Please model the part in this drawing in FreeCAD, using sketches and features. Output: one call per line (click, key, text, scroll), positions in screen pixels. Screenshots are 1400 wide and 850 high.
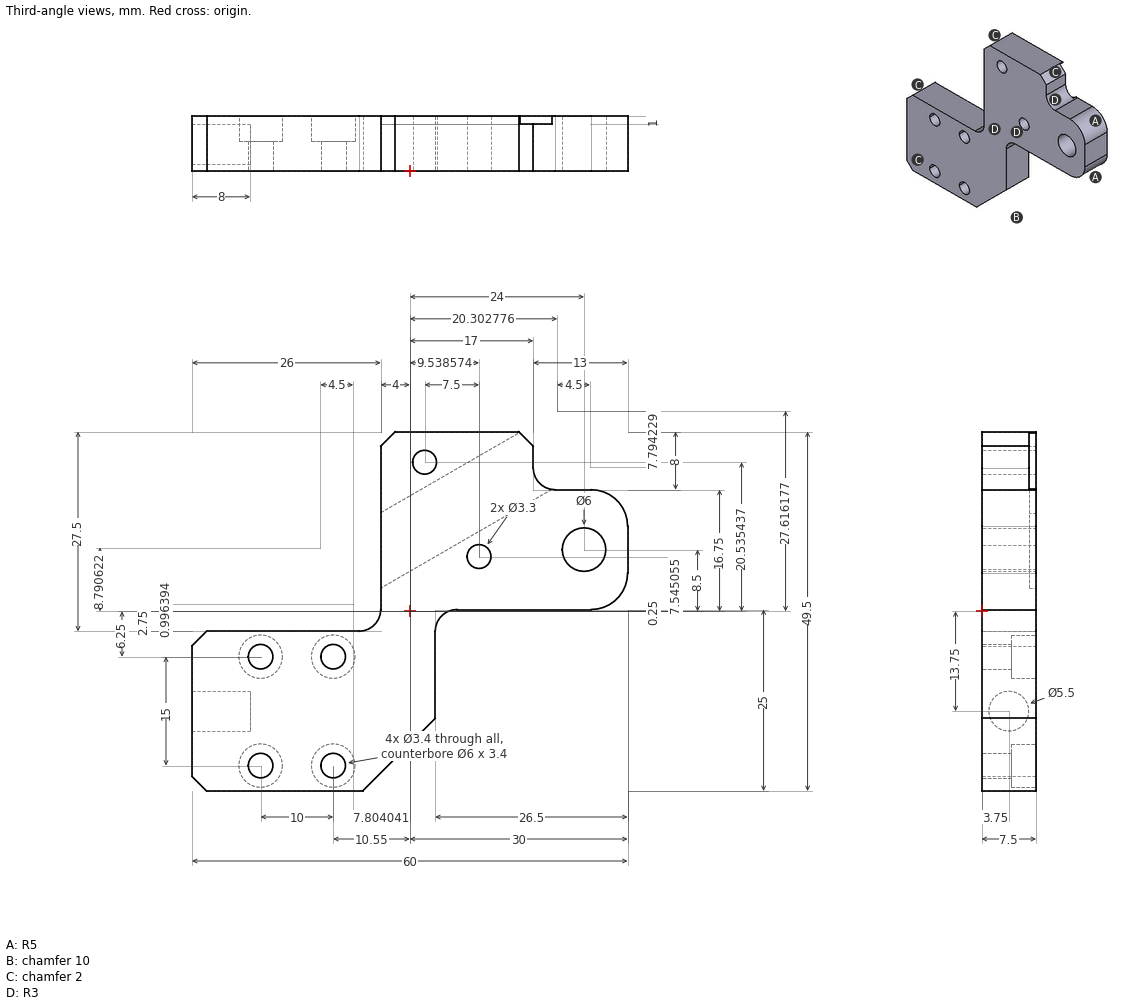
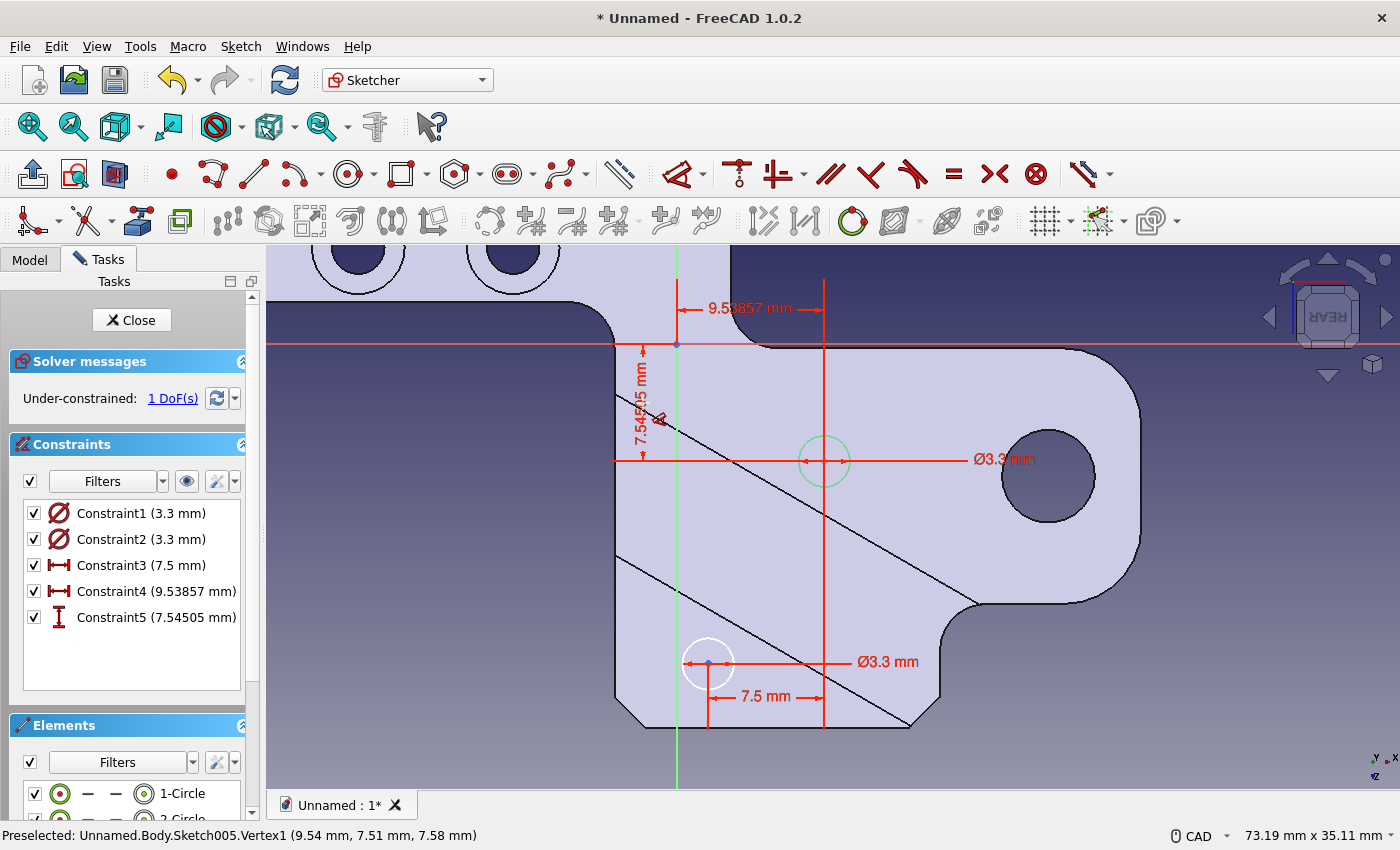
click(708, 664)
click(643, 504)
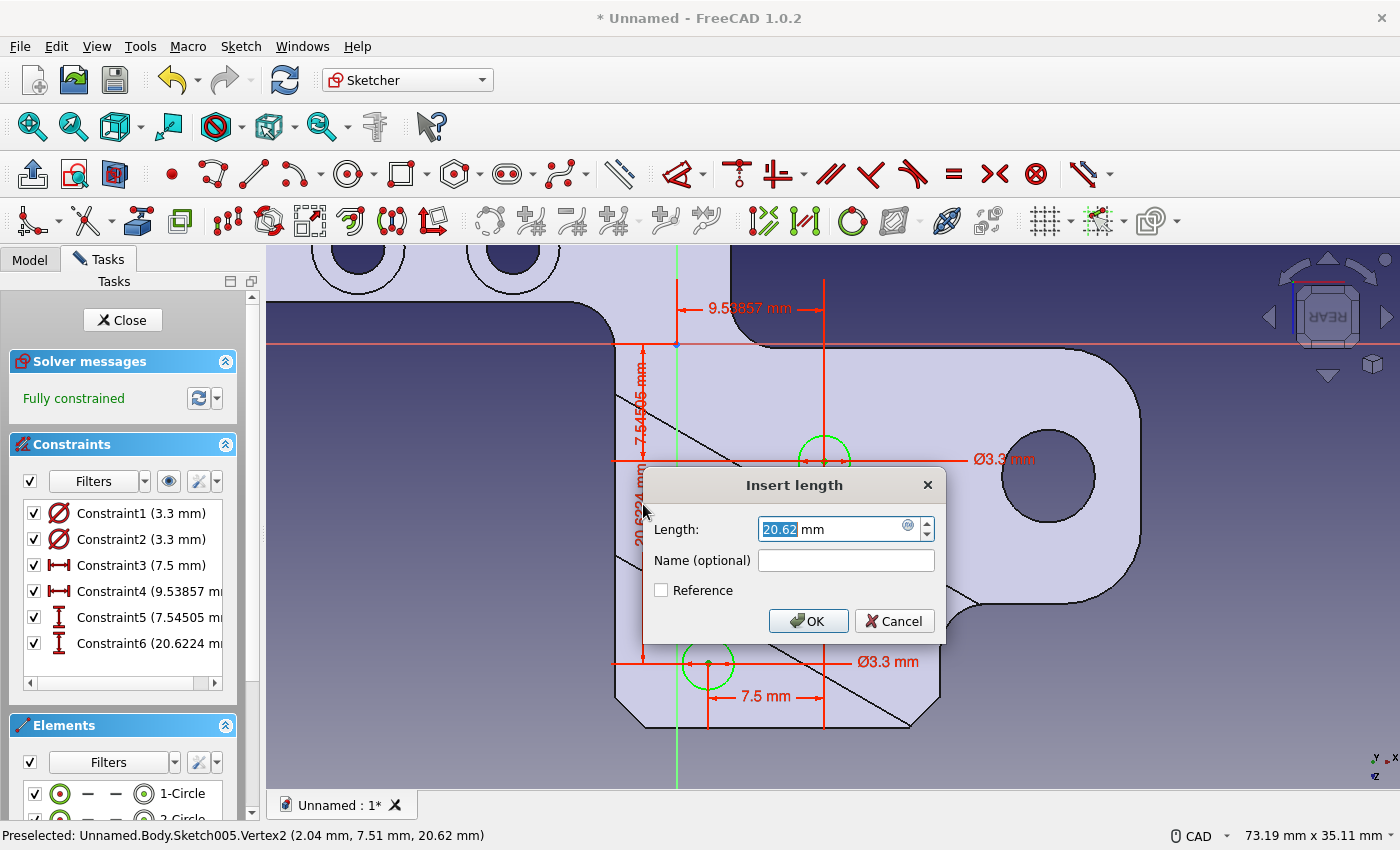
text(20.535437)
key(Return)
key(Escape)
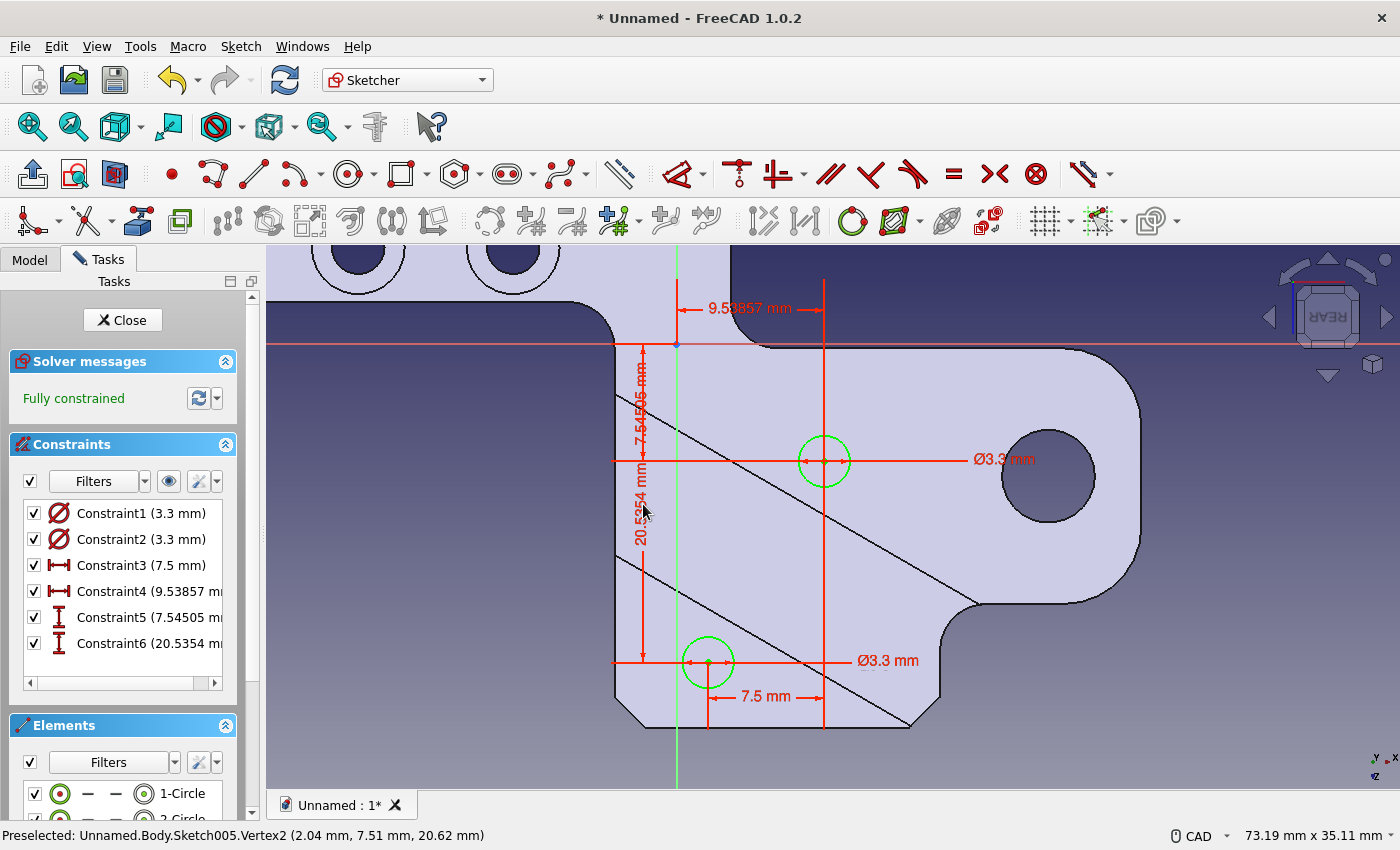
click(123, 320)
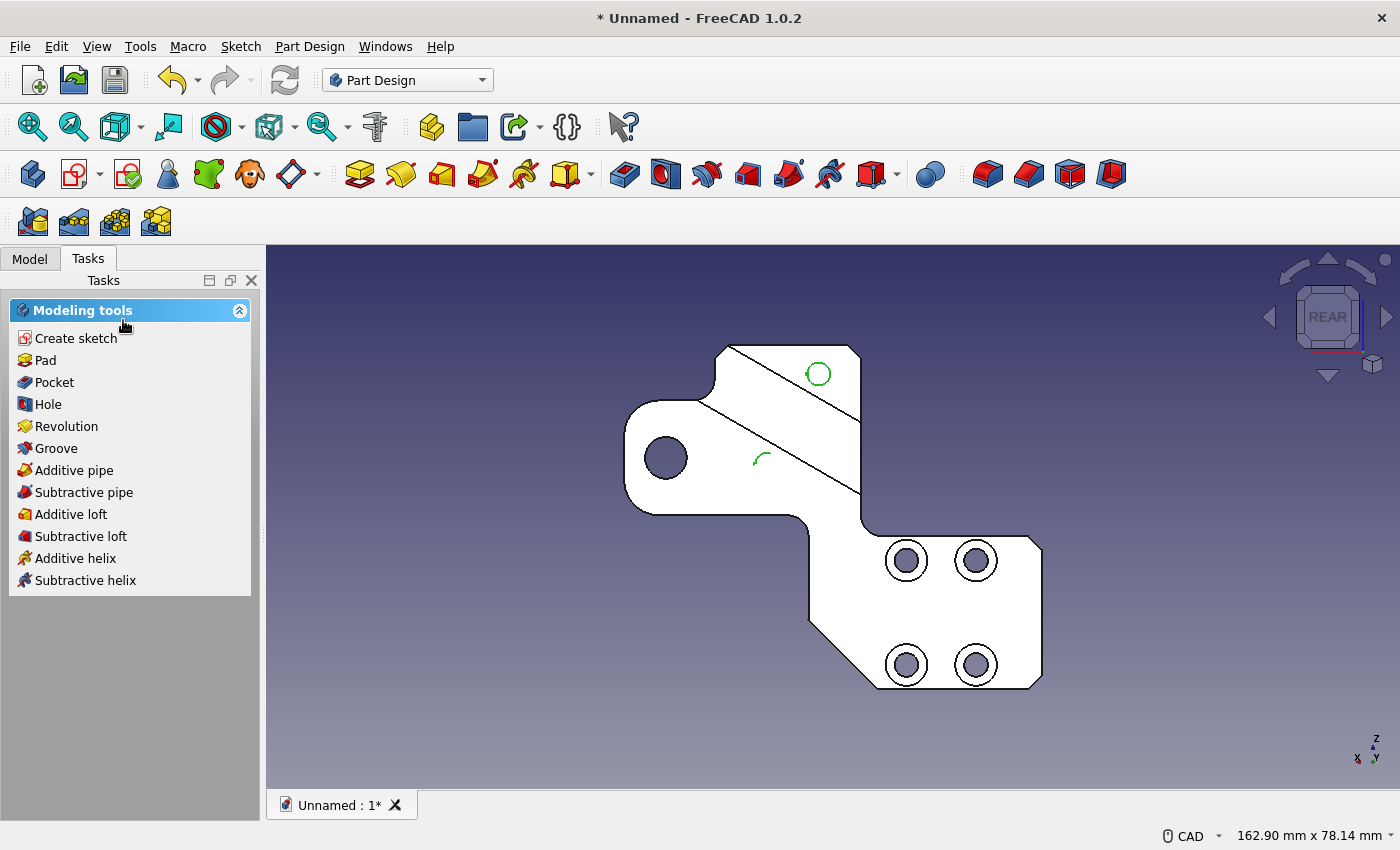
click(625, 174)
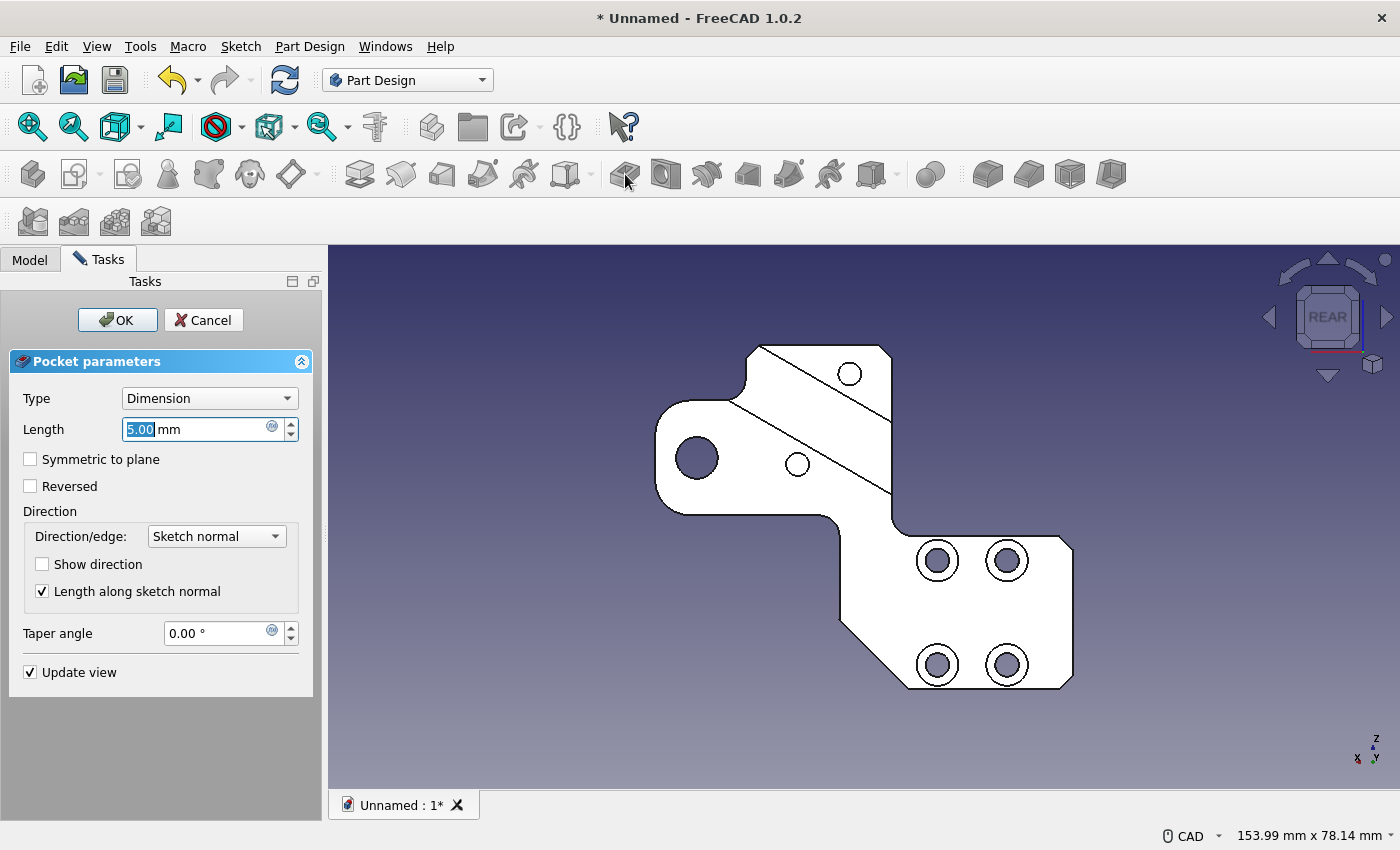
click(210, 398)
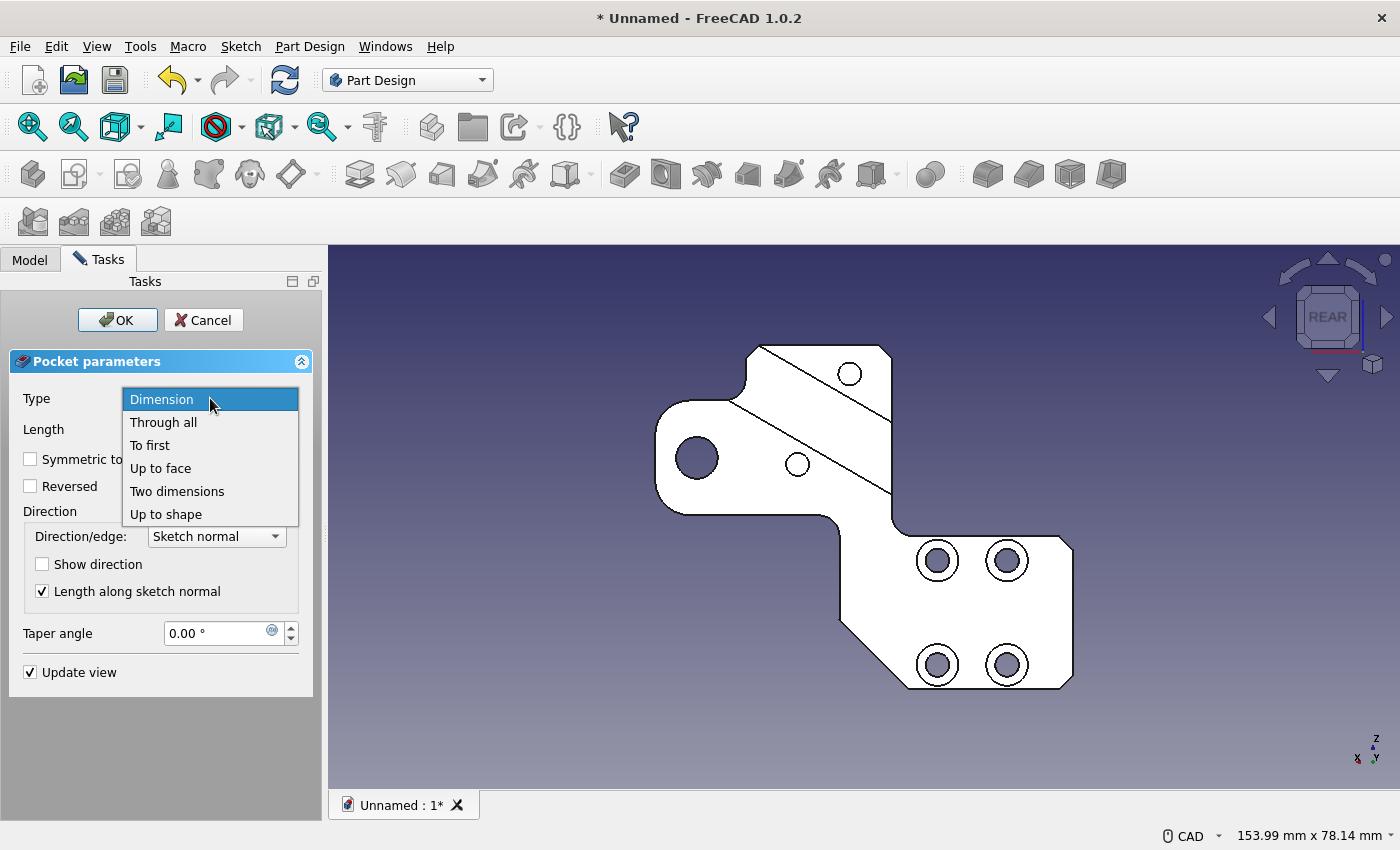
click(208, 422)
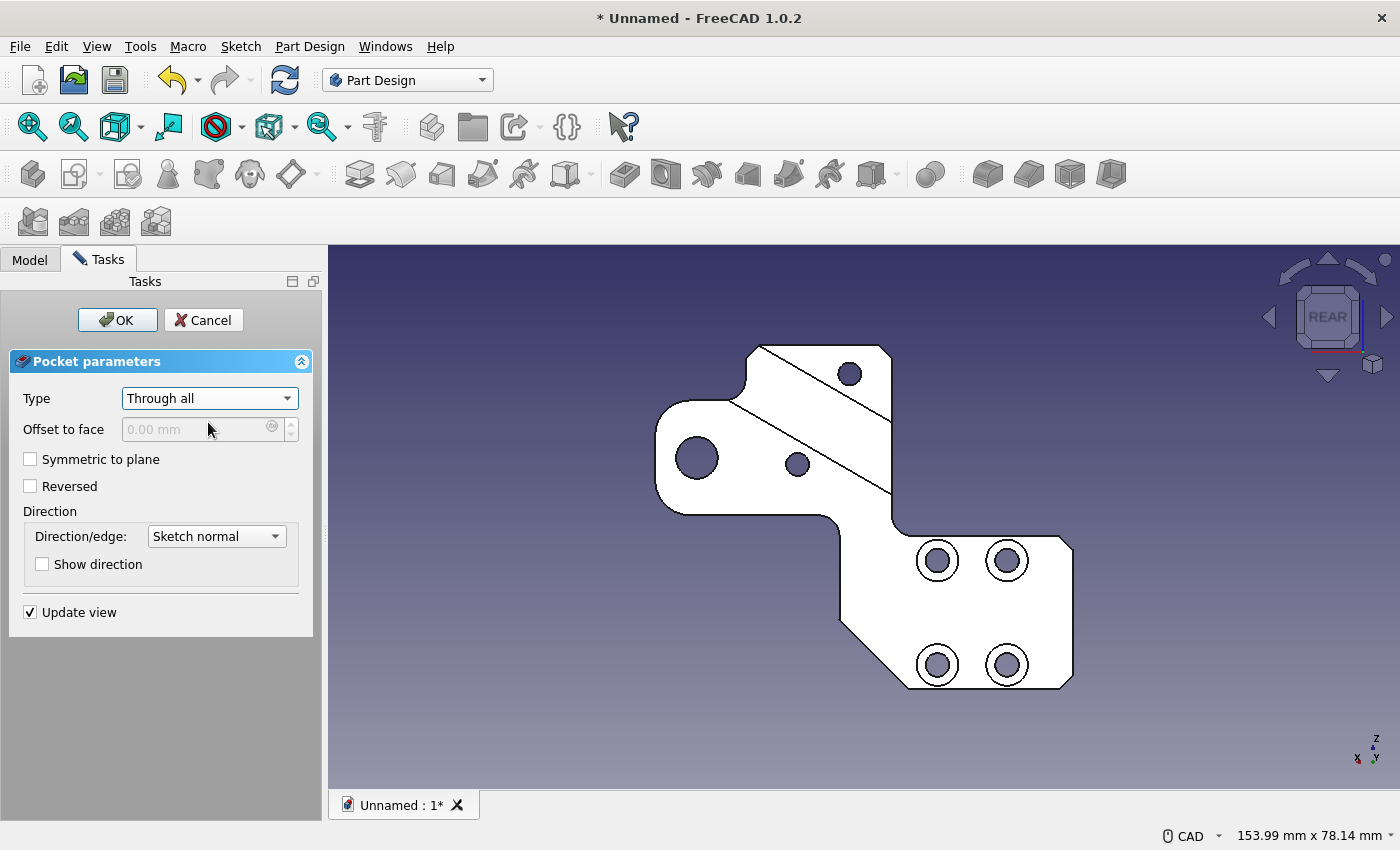
click(118, 320)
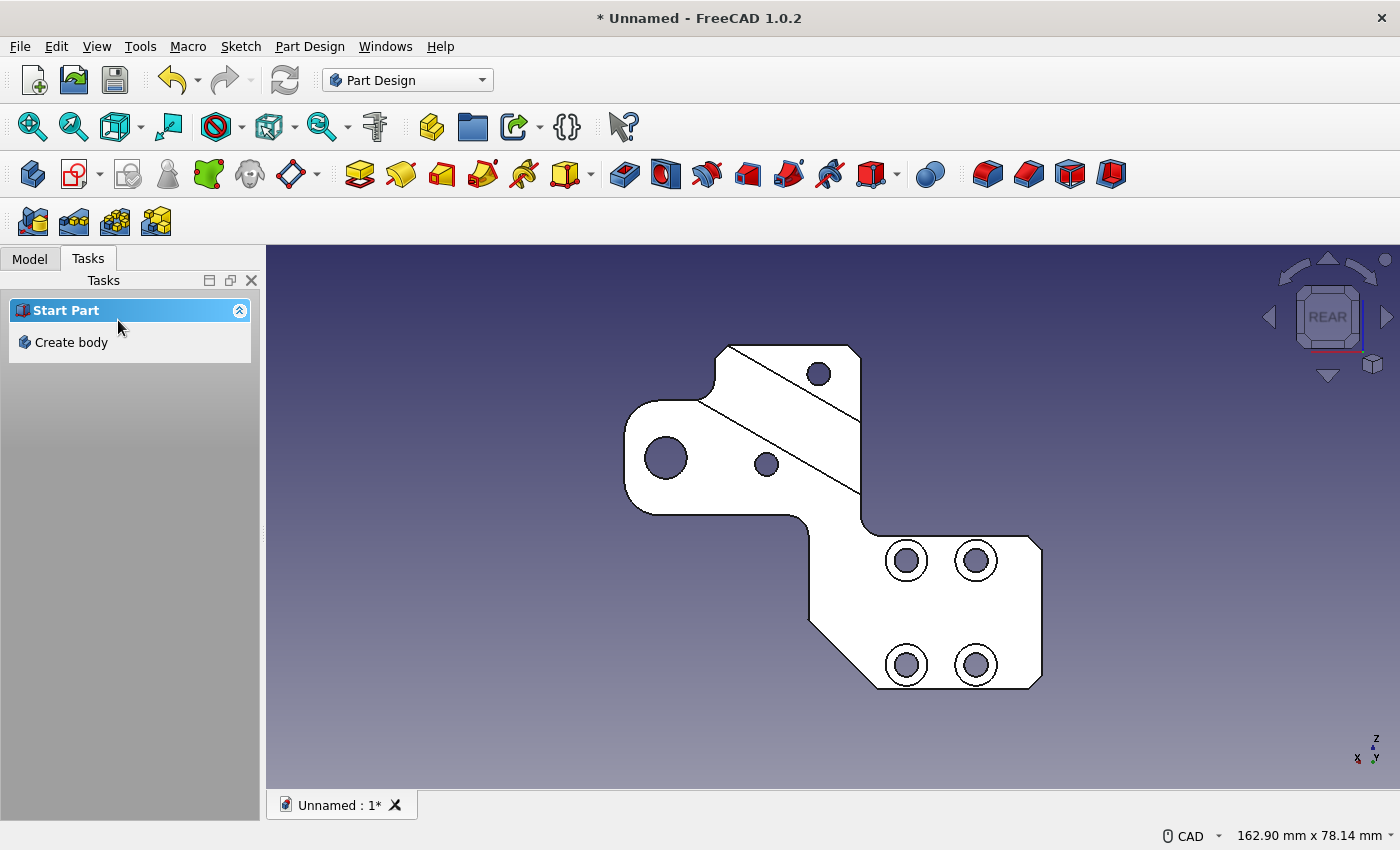
key(6)